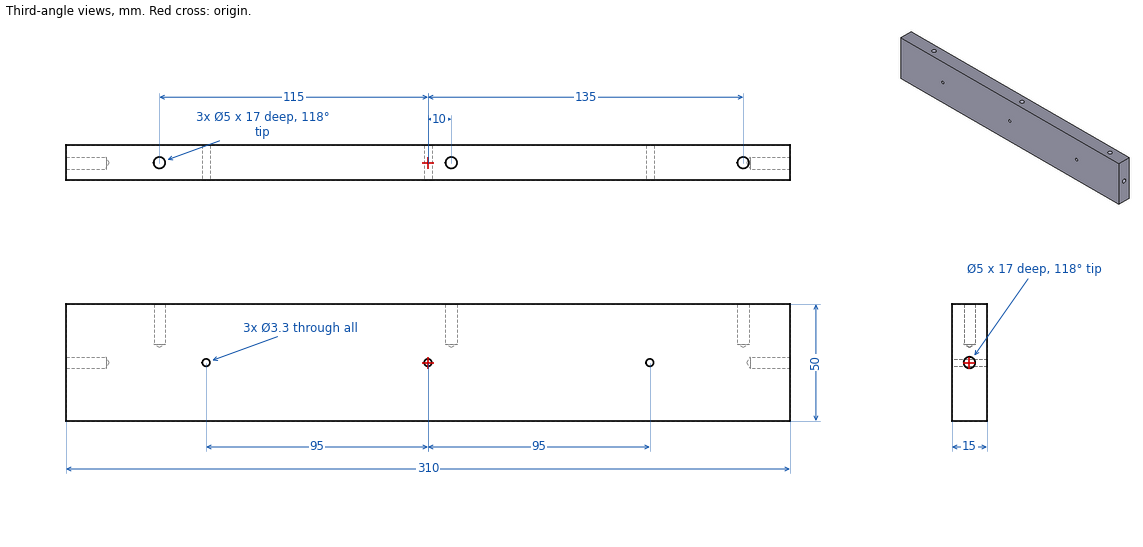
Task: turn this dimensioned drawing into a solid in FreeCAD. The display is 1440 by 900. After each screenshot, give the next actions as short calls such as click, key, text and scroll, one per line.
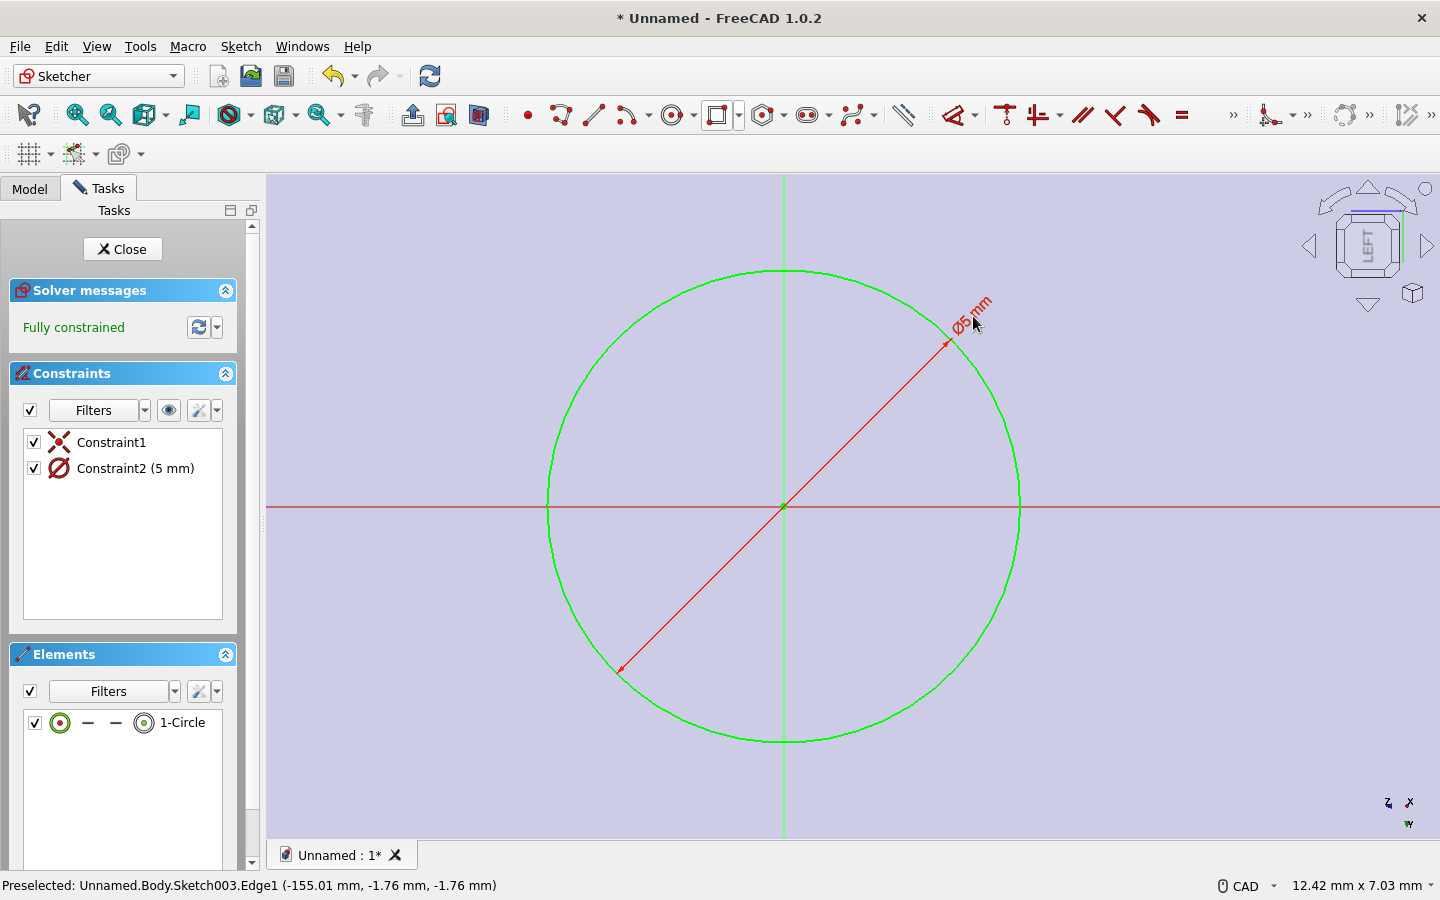
click(123, 249)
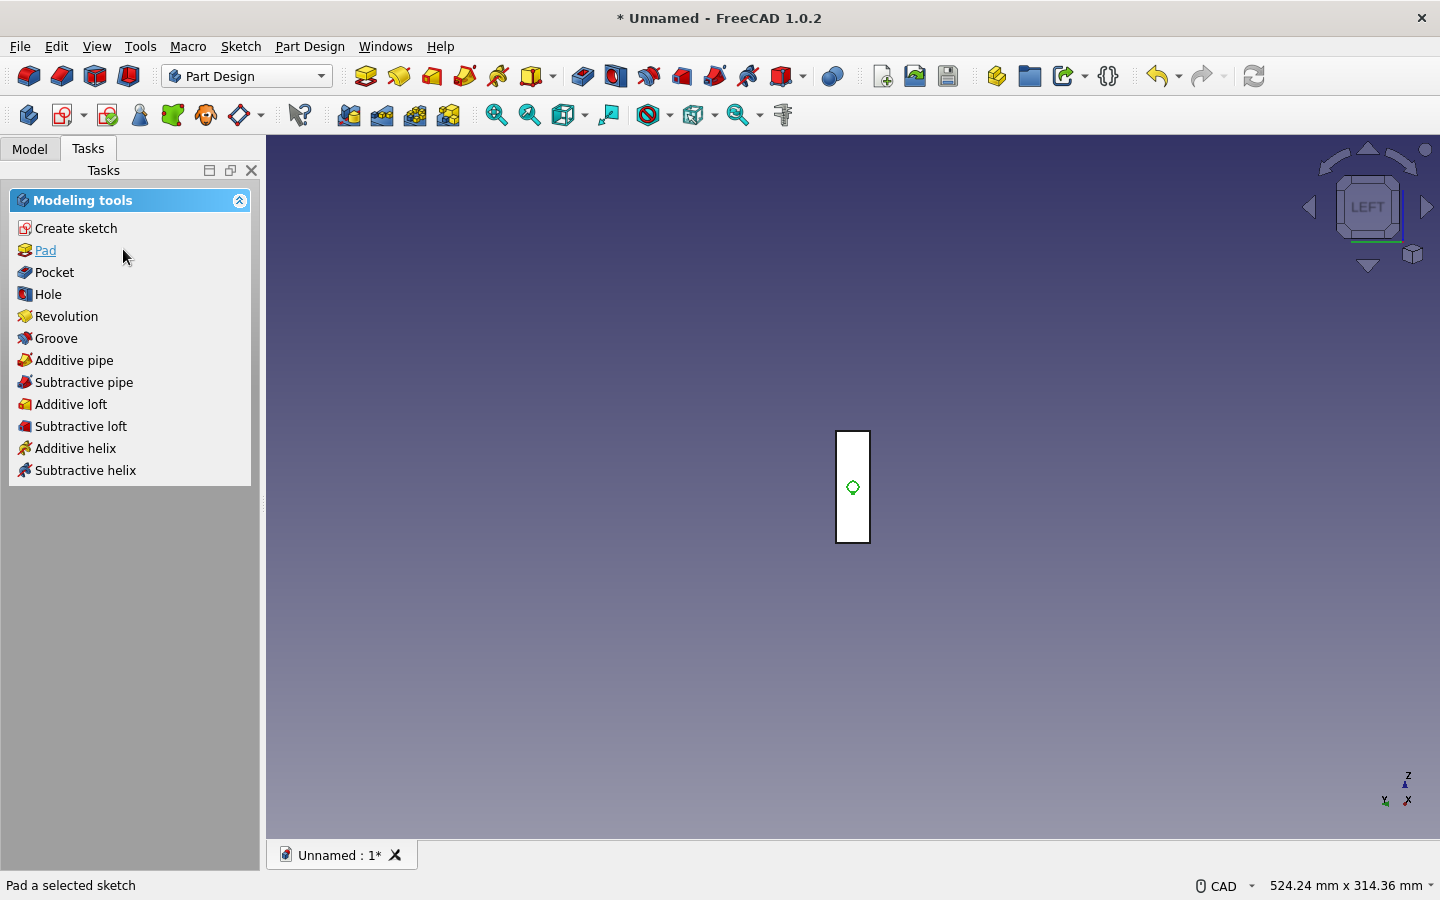
click(616, 76)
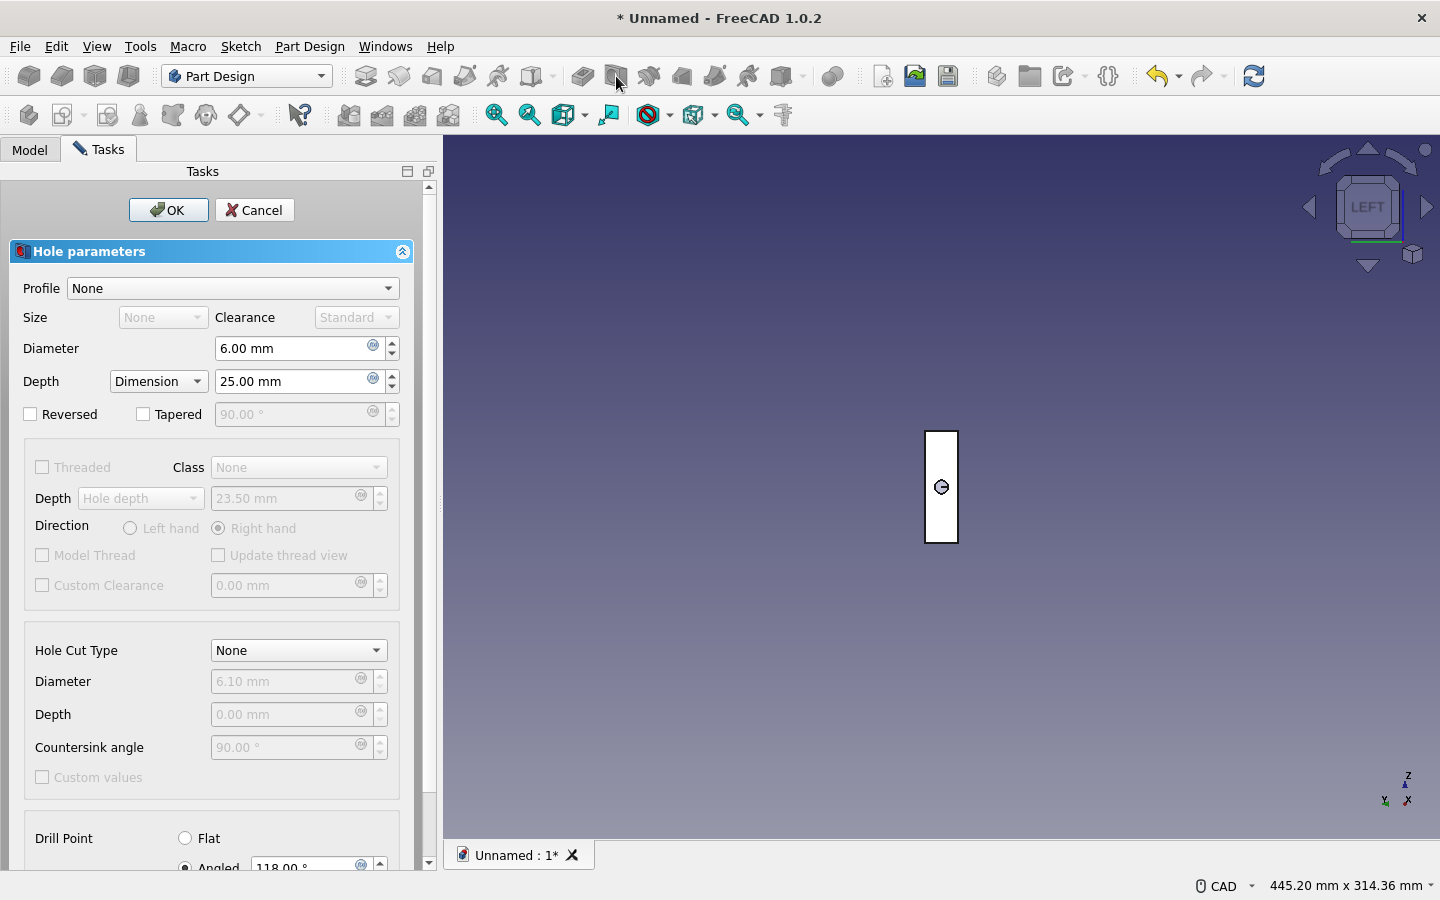
triple_click(300, 348)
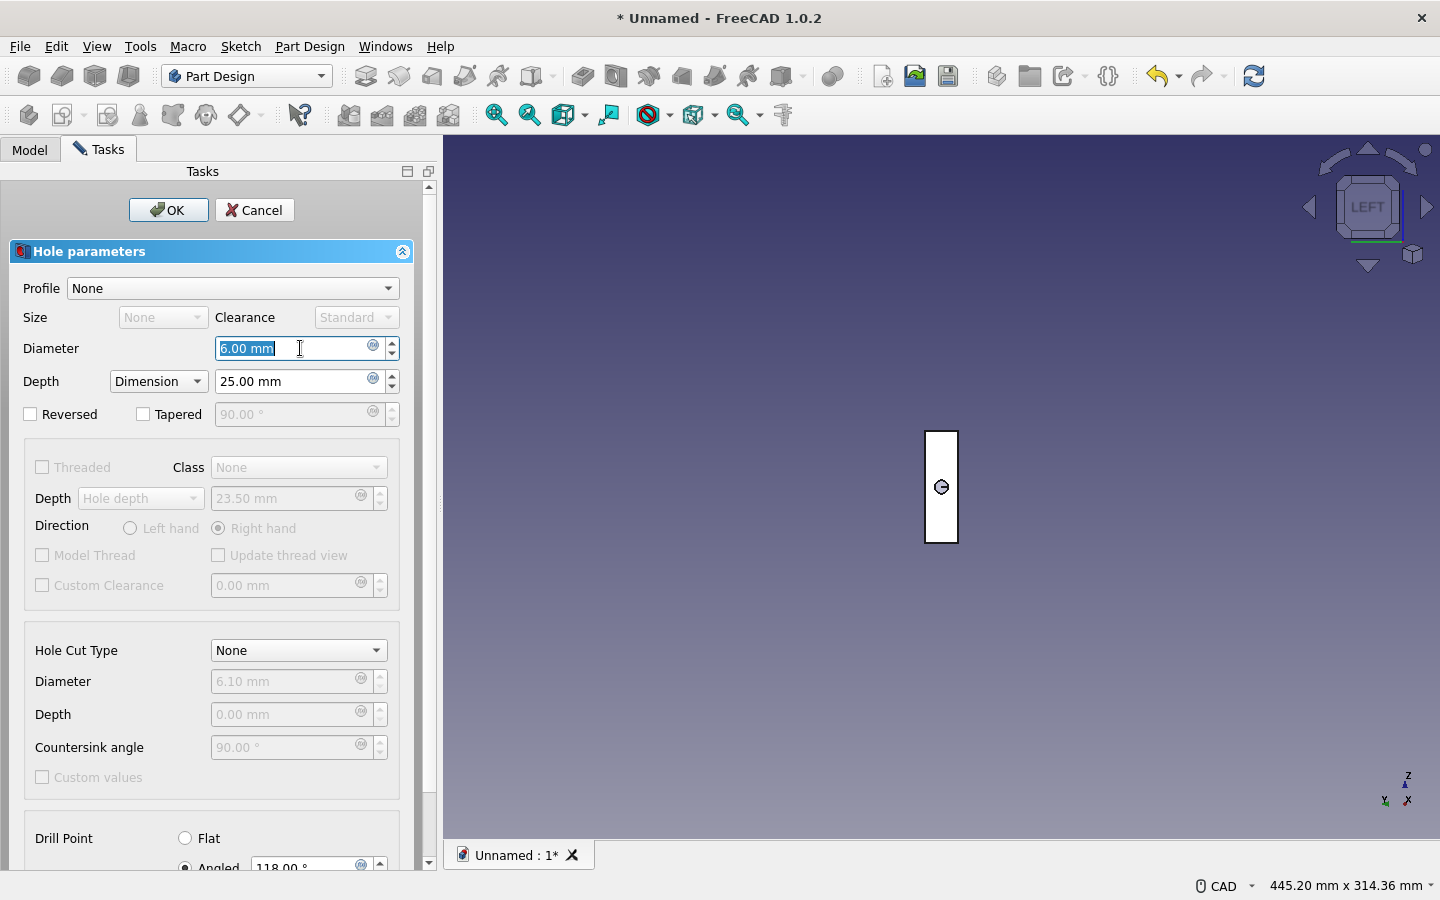
text(5)
key(Tab)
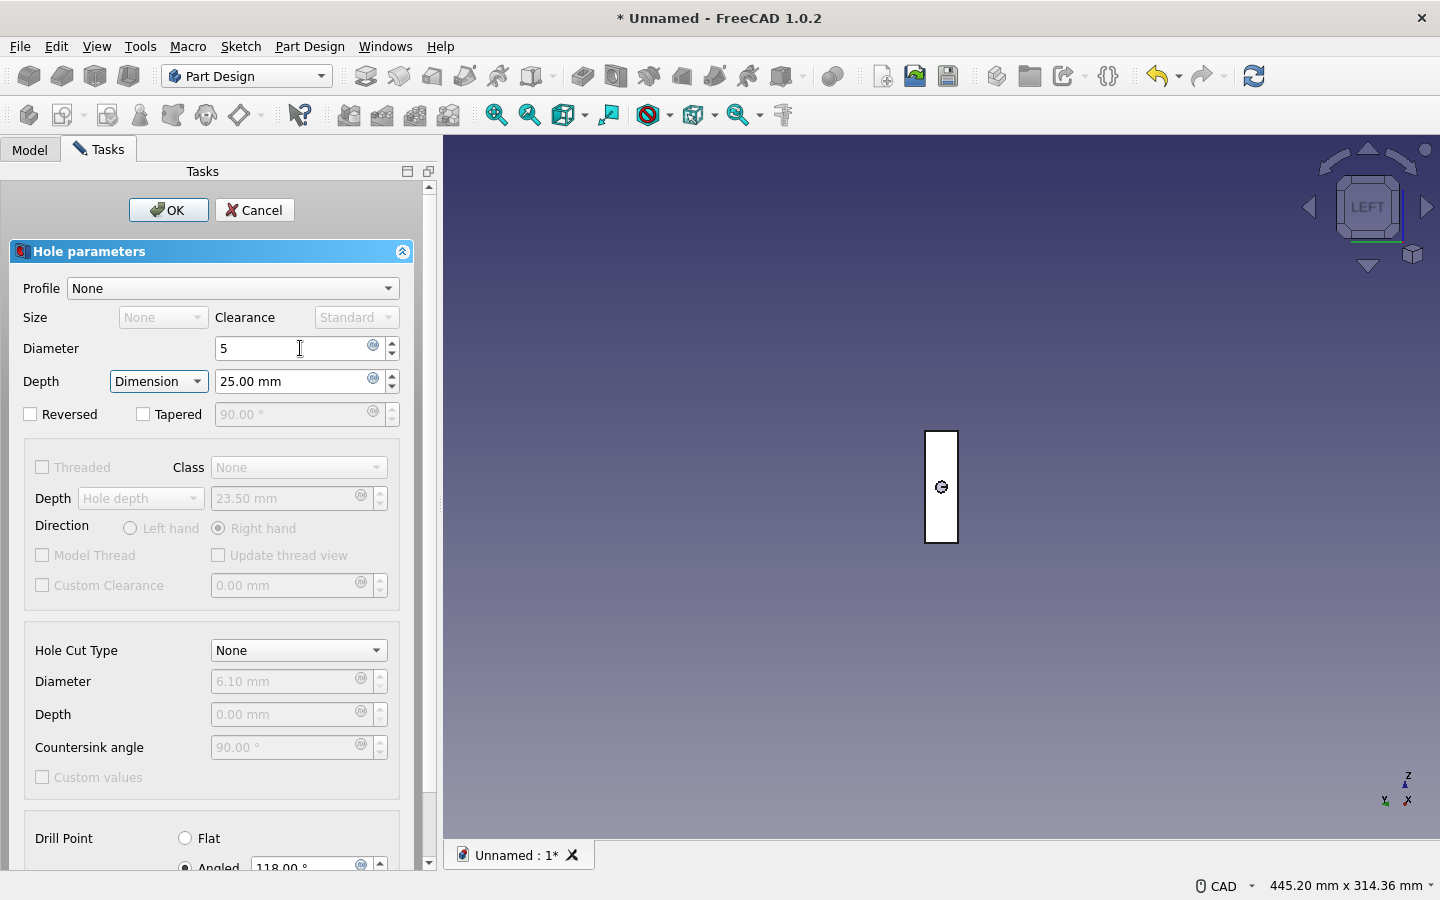
triple_click(300, 382)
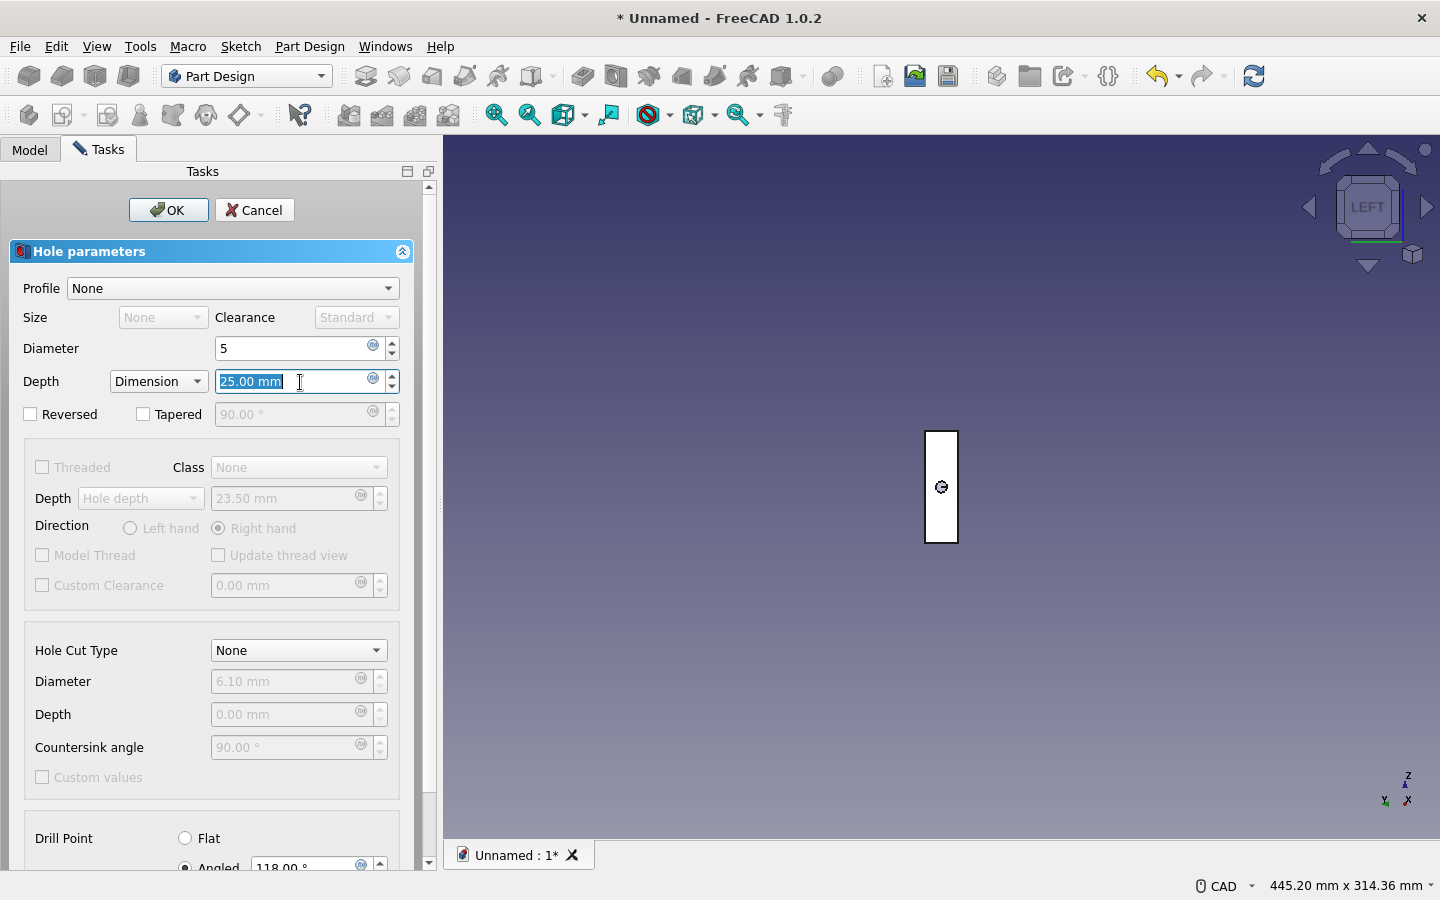
text(17)
key(Tab)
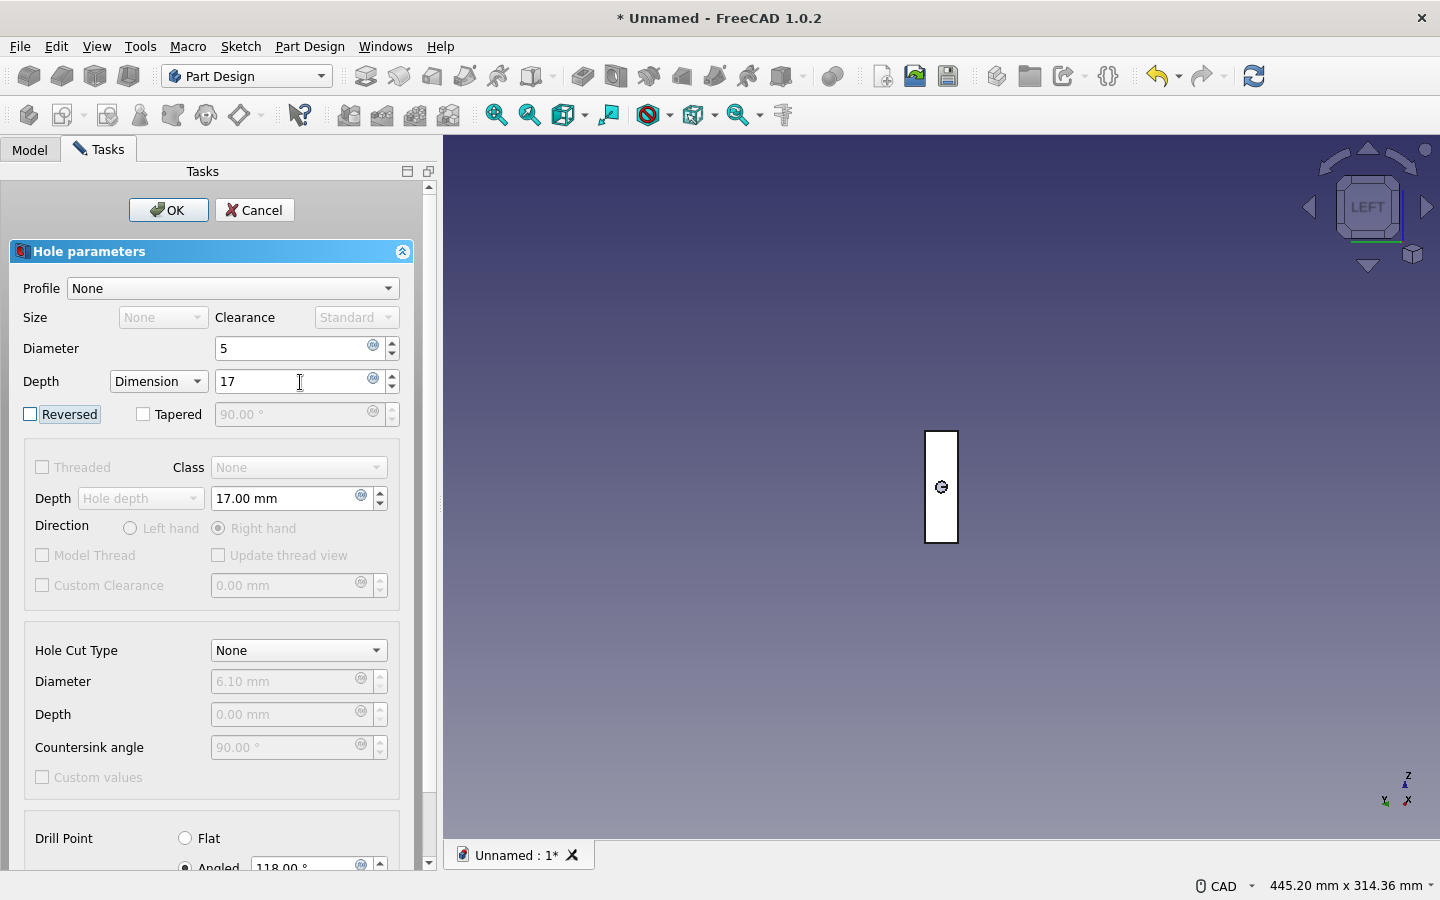
click(169, 210)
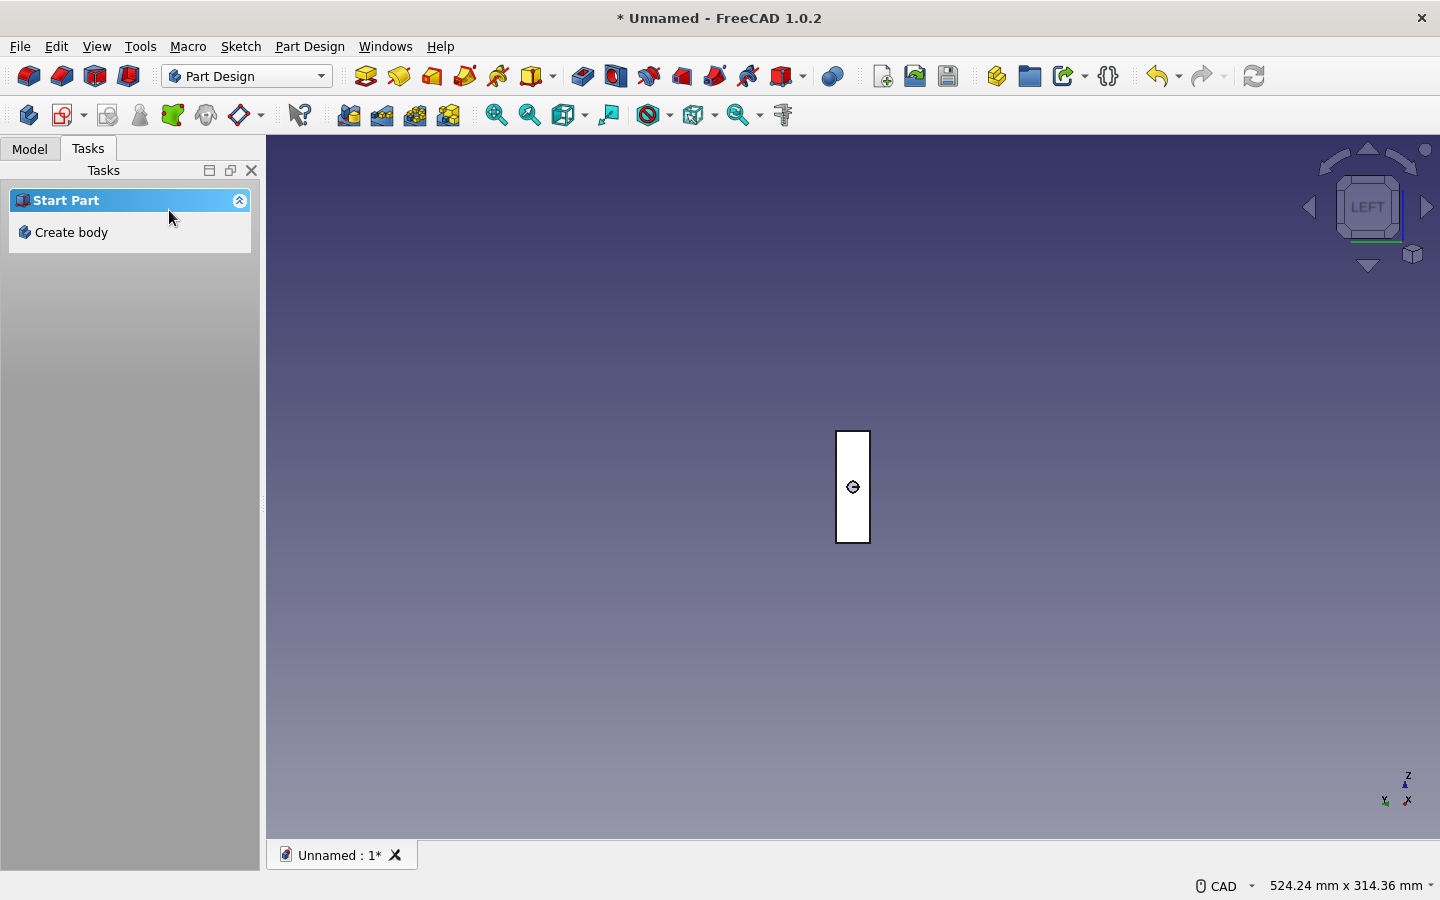
click(497, 116)